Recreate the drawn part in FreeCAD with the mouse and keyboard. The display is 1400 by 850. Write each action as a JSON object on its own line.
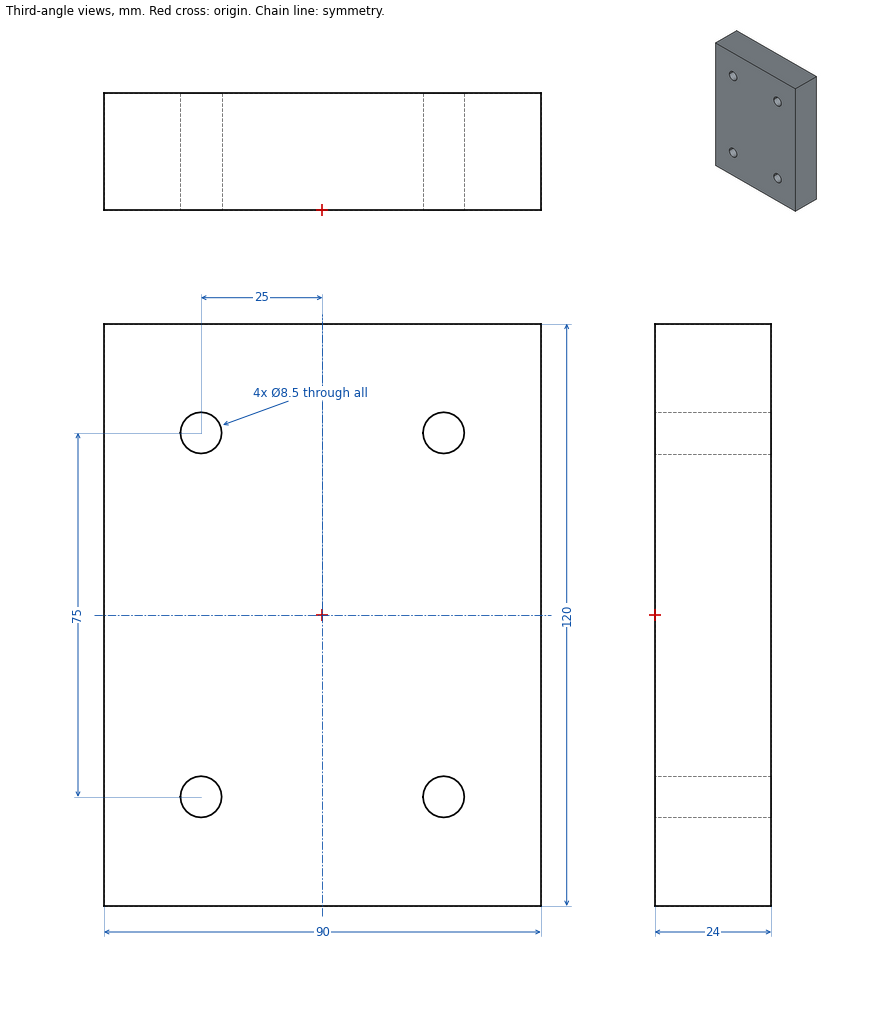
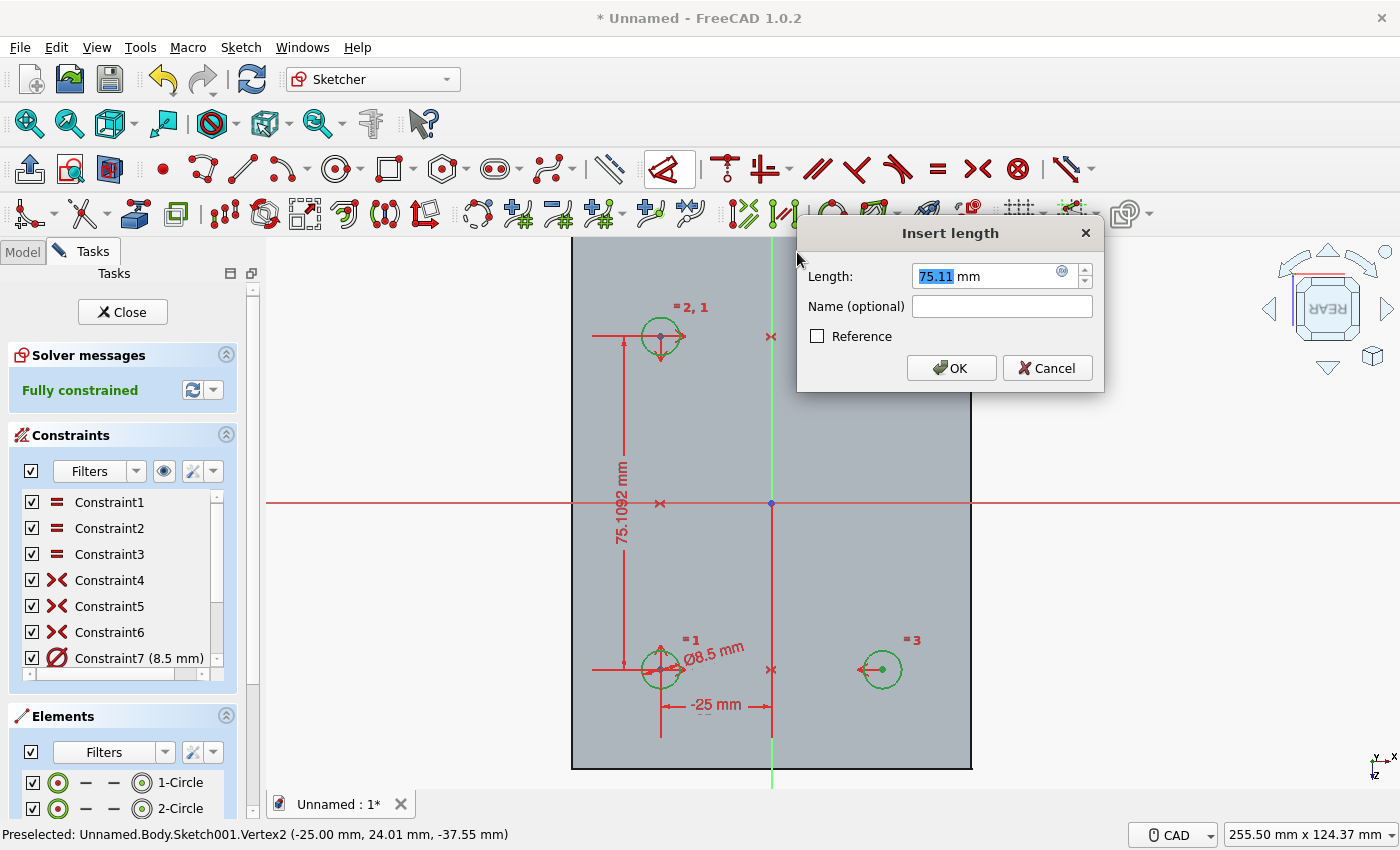
{"action": "type", "text": "75"}
{"action": "key", "text": "Return"}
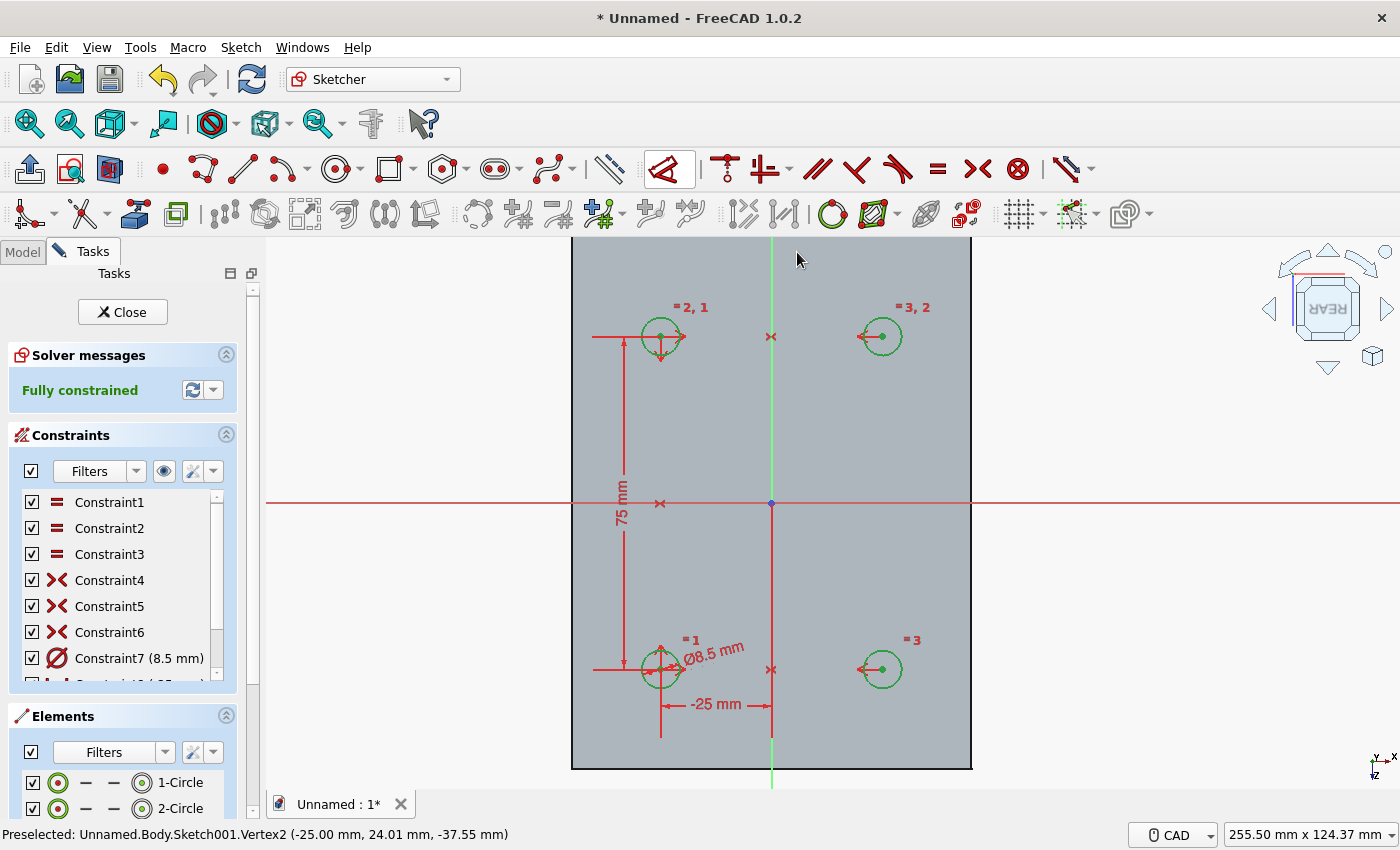
{"action": "left_click", "coordinate": [123, 312]}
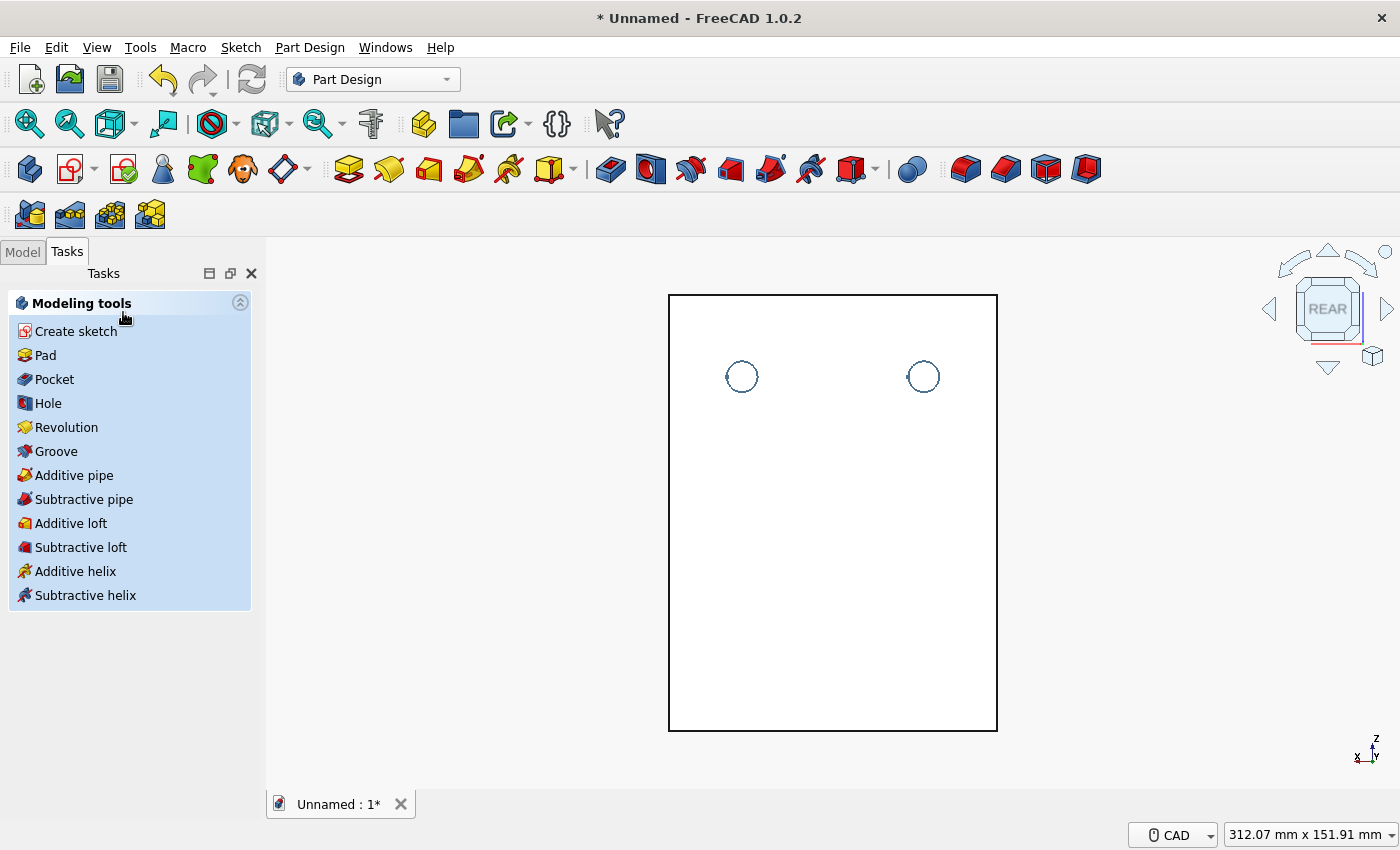
{"action": "left_click", "coordinate": [652, 170]}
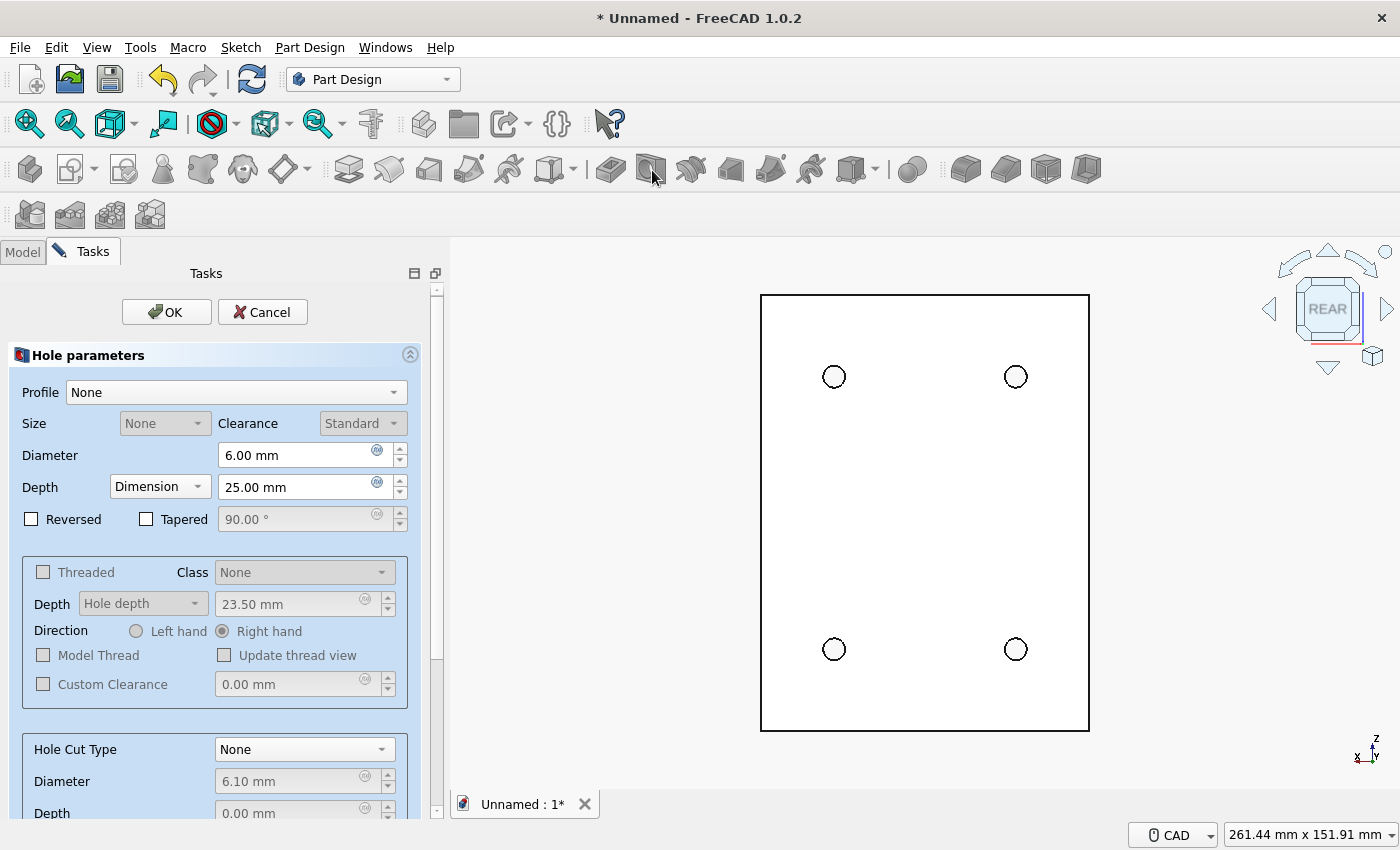
{"action": "triple_click", "coordinate": [305, 455]}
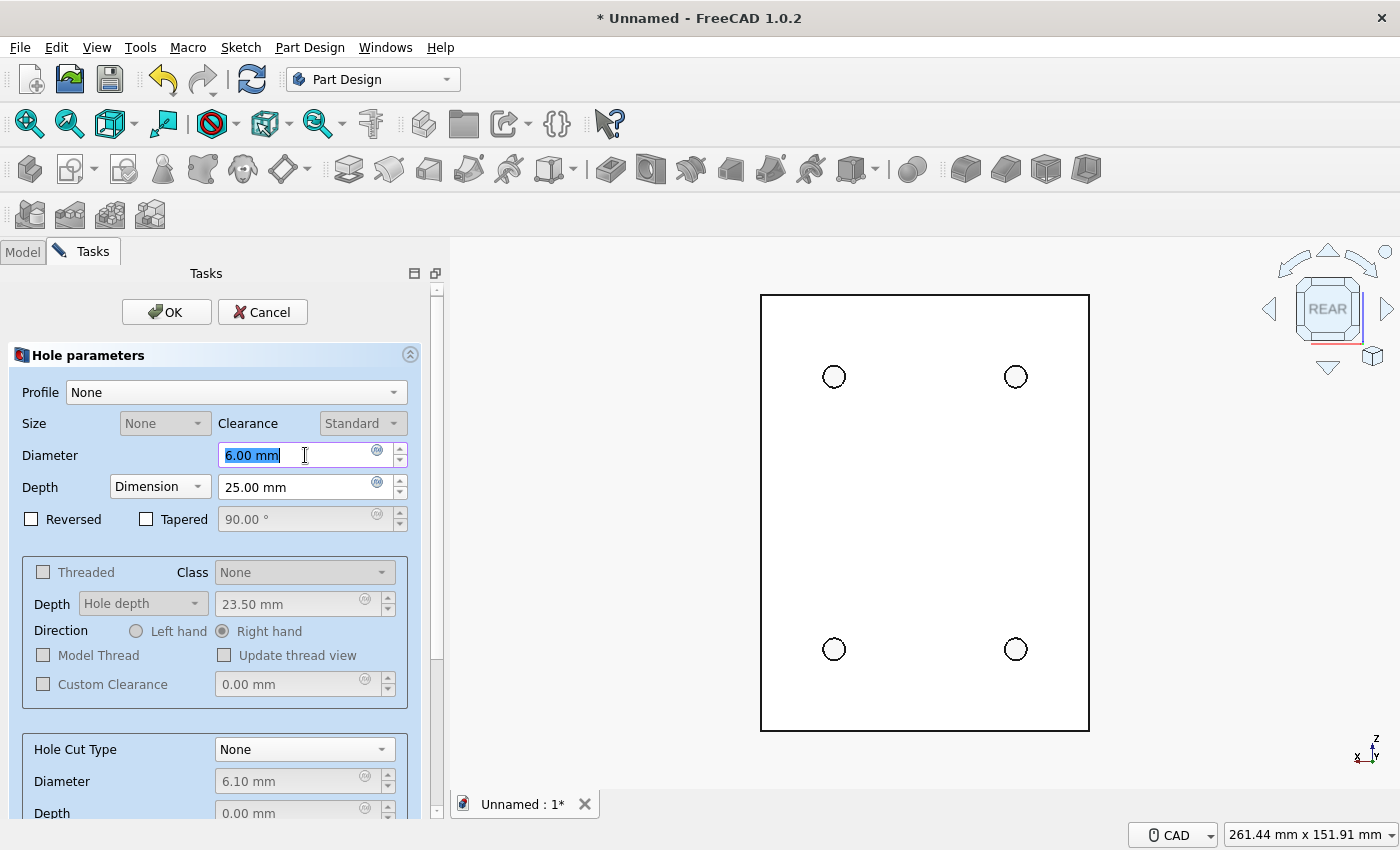
{"action": "type", "text": "8.5"}
{"action": "key", "text": "Tab"}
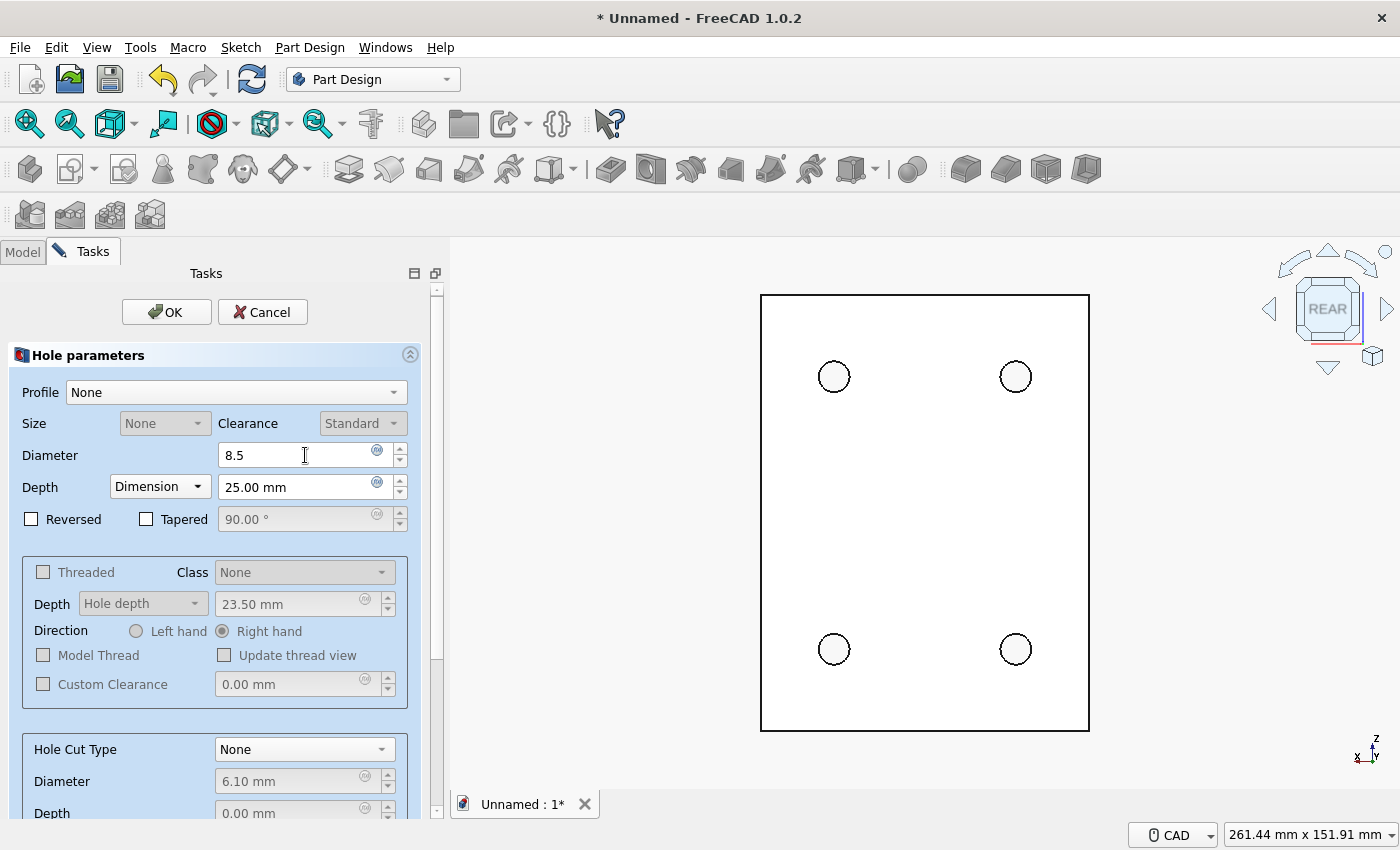
{"action": "left_click", "coordinate": [161, 486]}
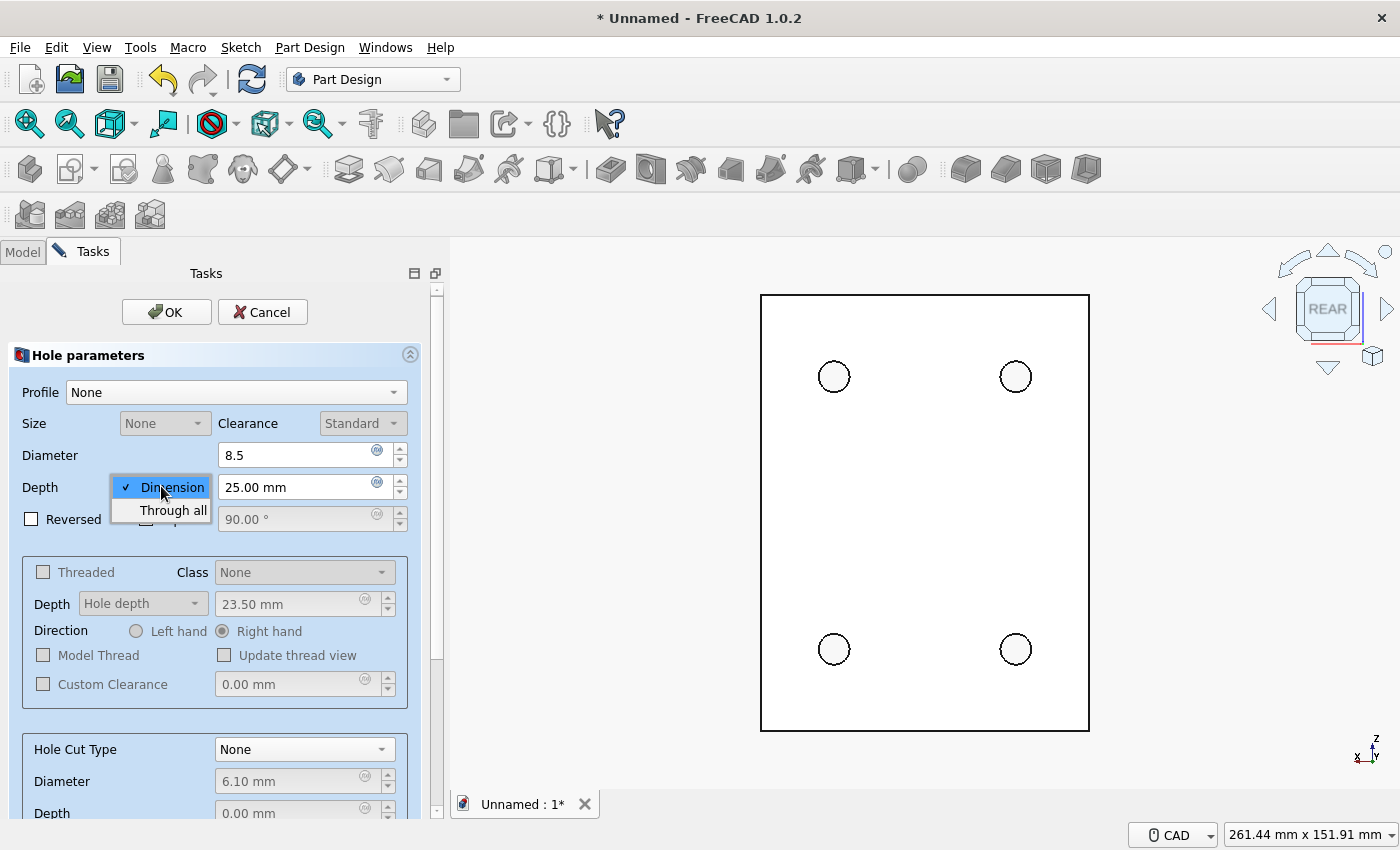
{"action": "left_click", "coordinate": [160, 510]}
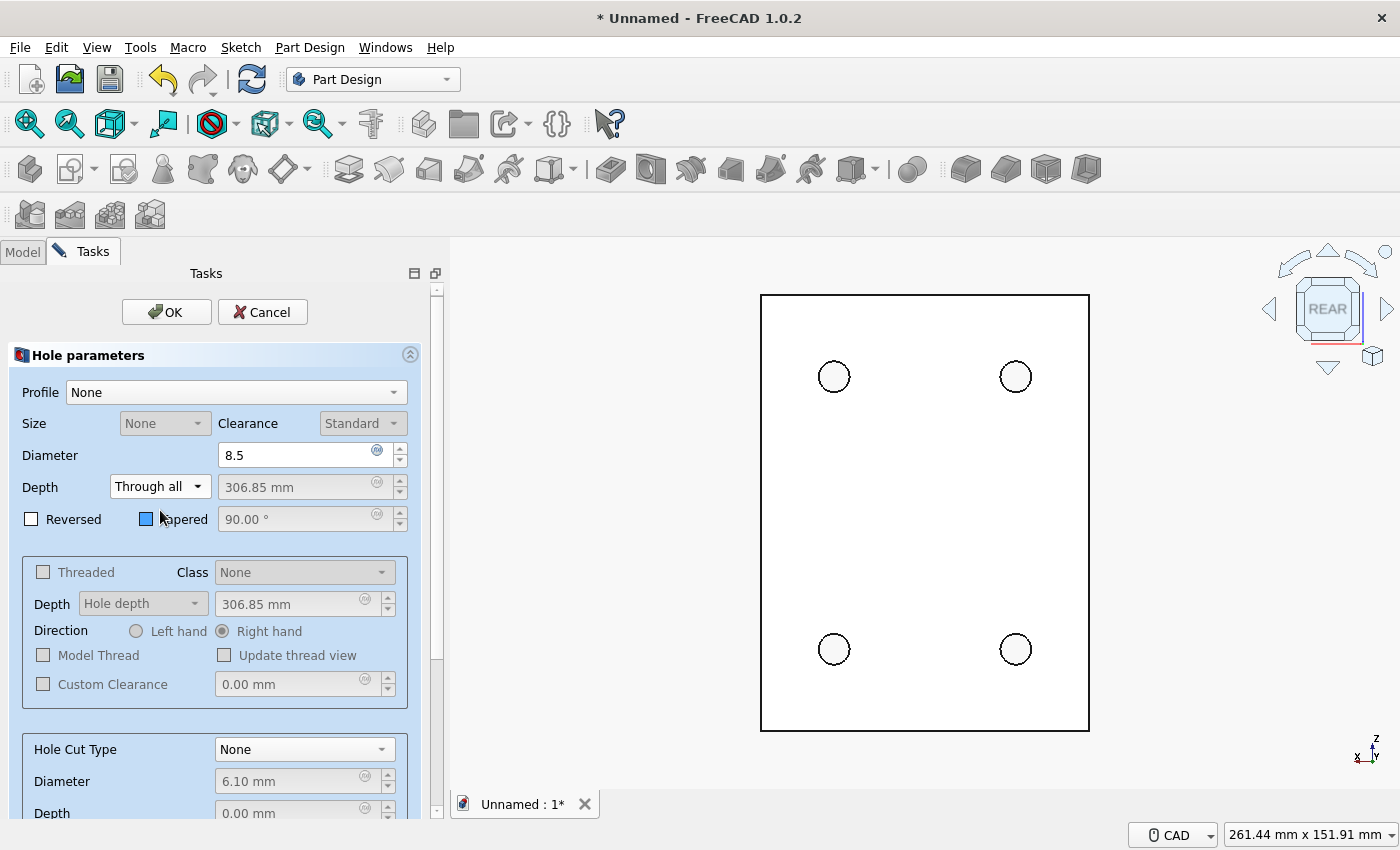
{"action": "left_click", "coordinate": [167, 312]}